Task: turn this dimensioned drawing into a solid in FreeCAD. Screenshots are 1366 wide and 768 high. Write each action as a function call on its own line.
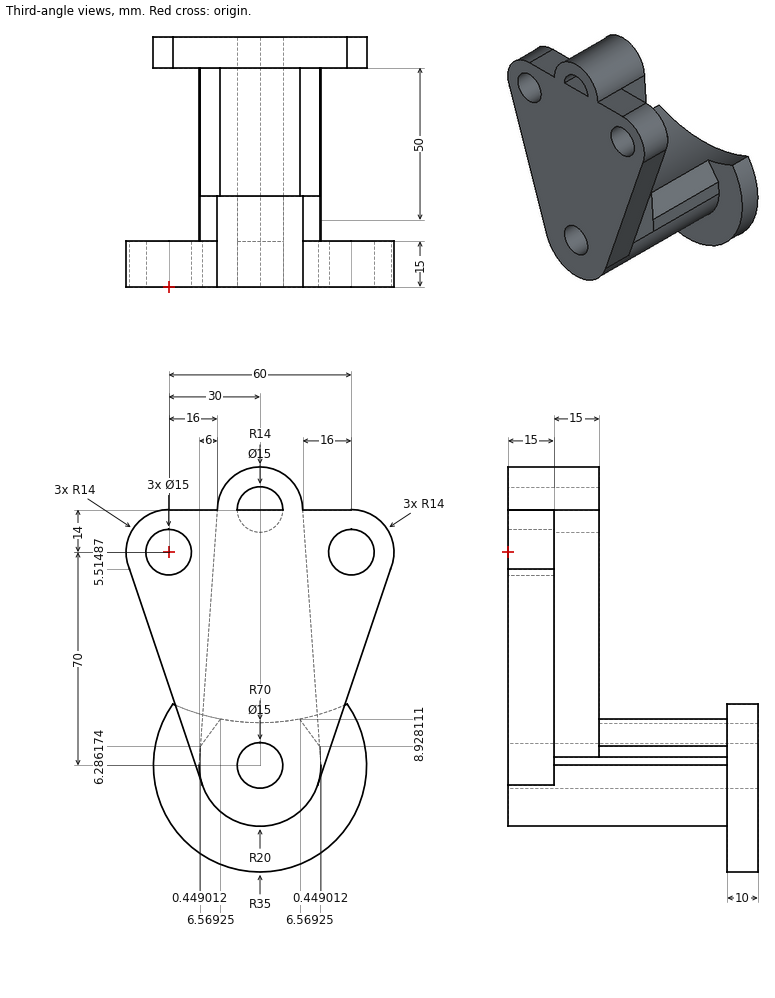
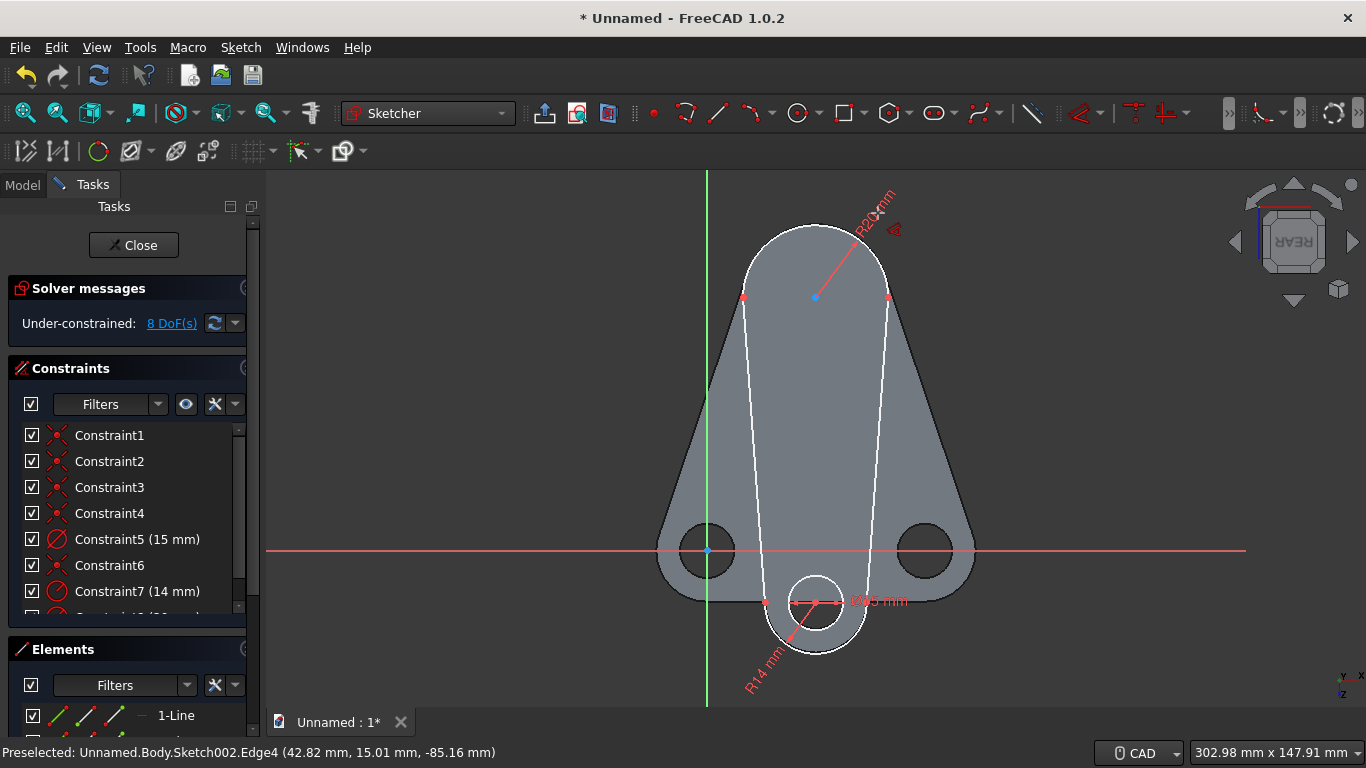
scroll(750, 390, up, 4)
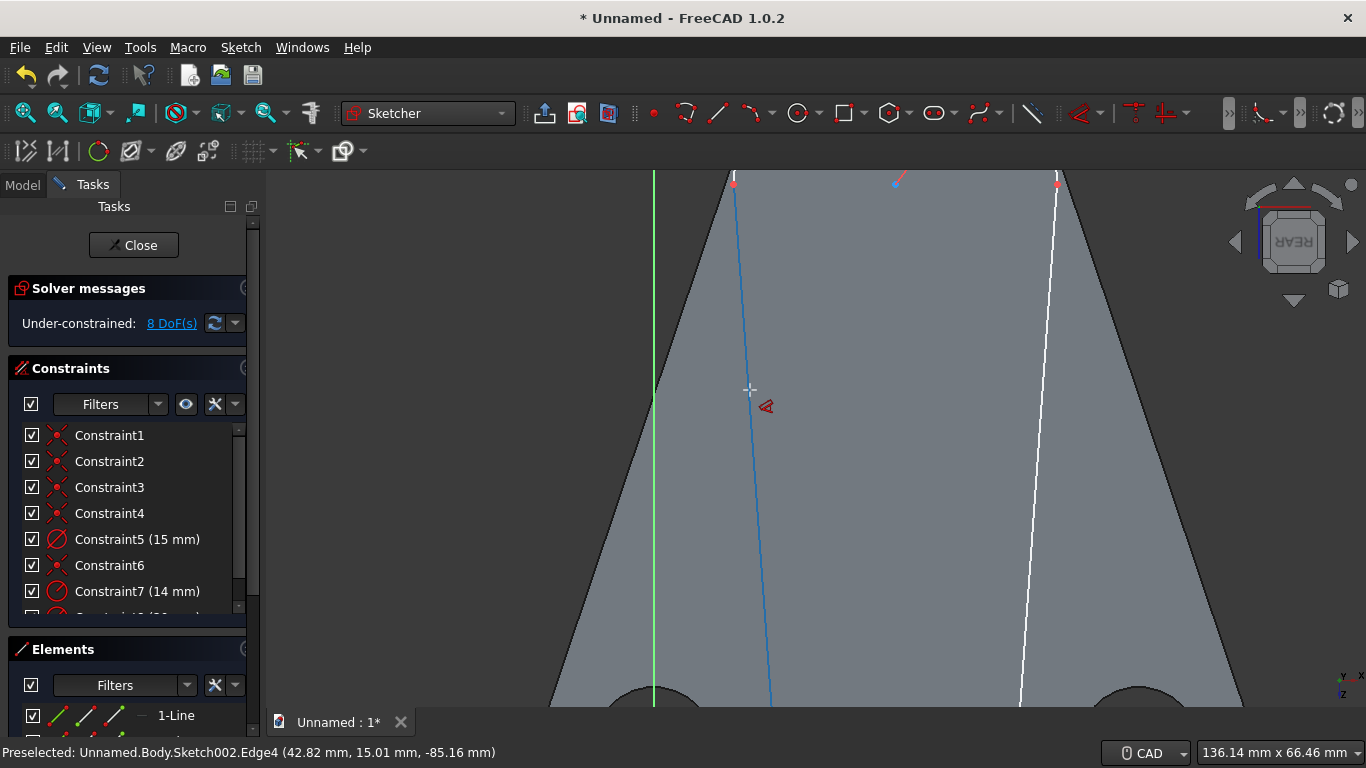
click(749, 388)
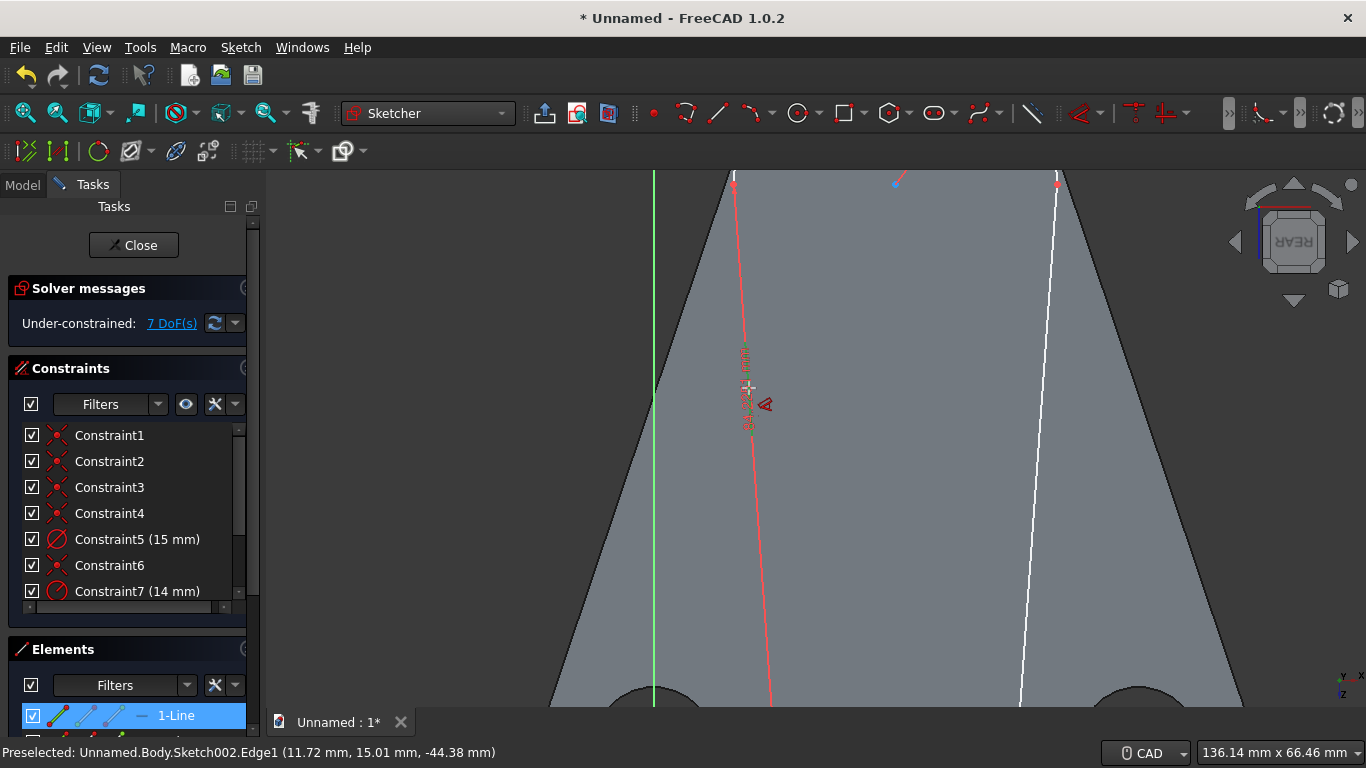
key(Escape)
key(Escape)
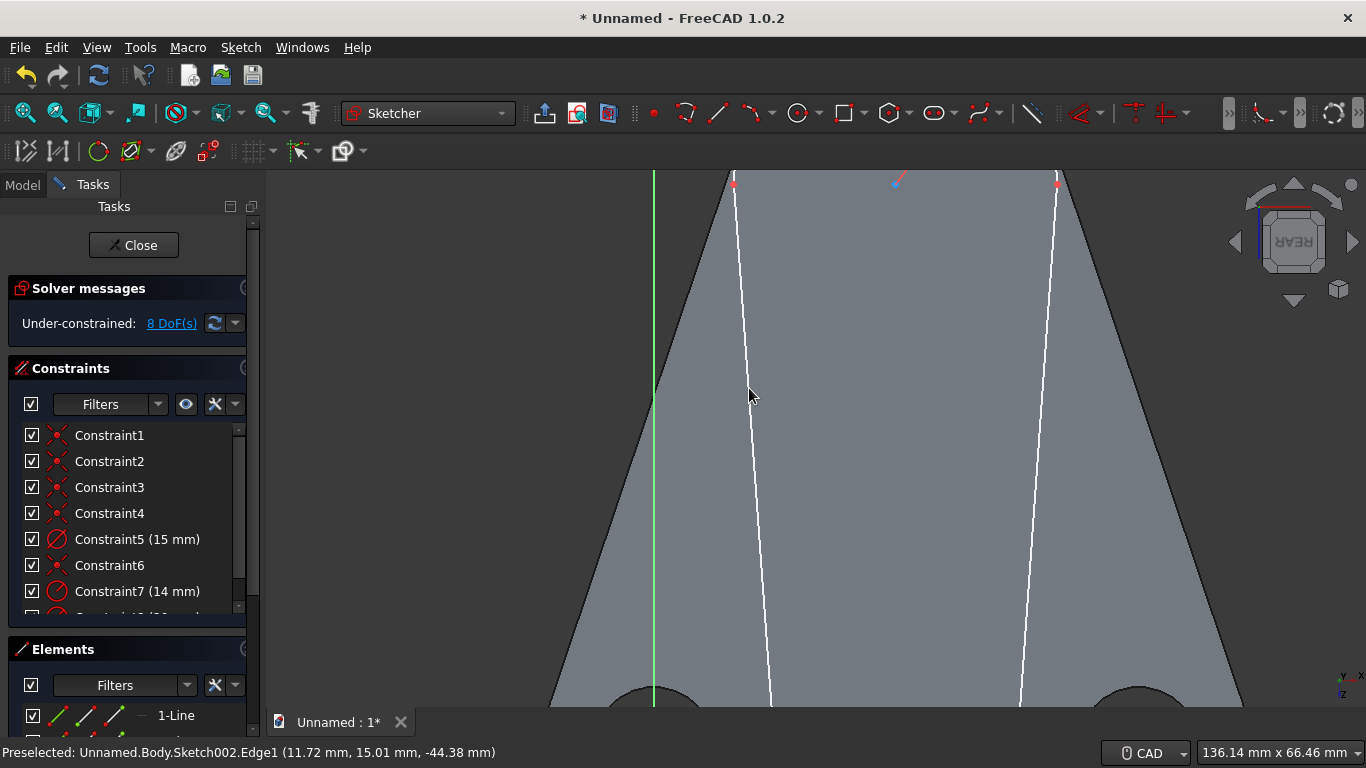
click(749, 388)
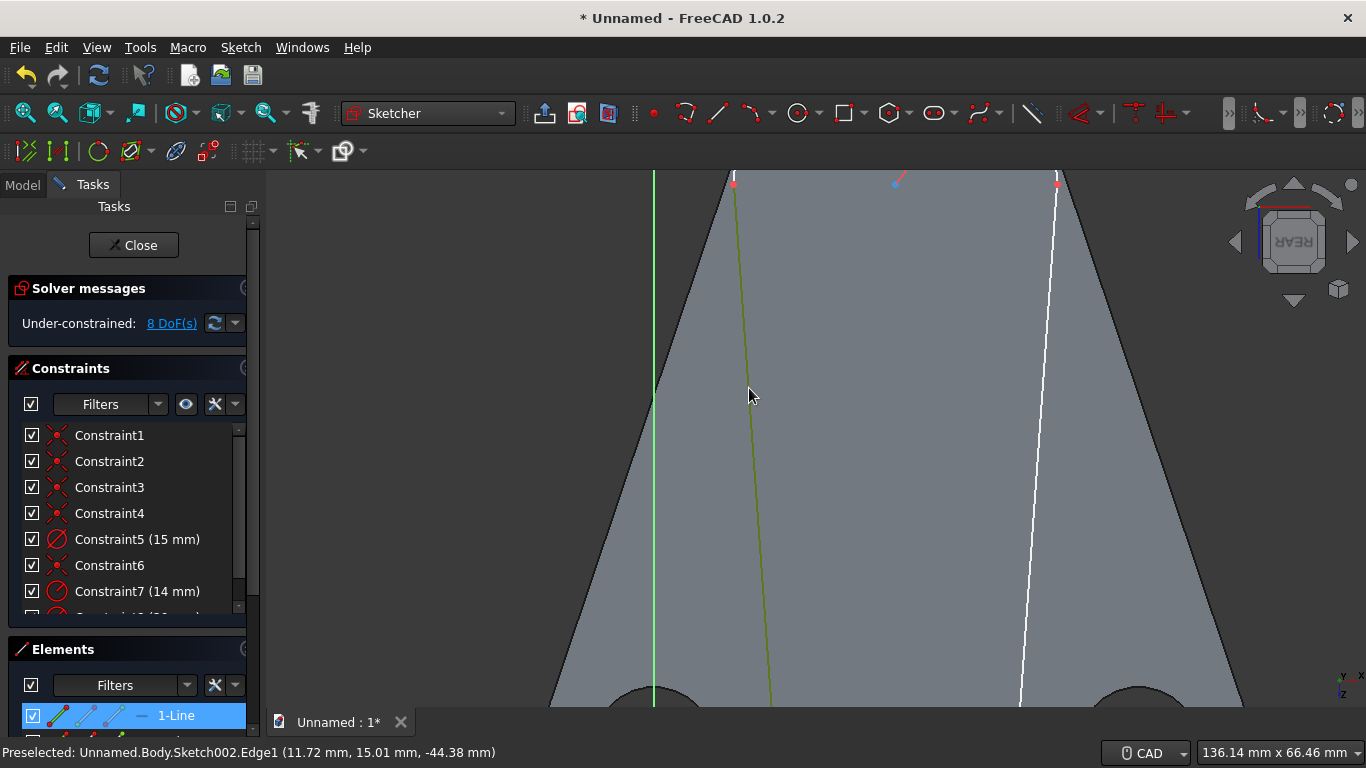
key(l)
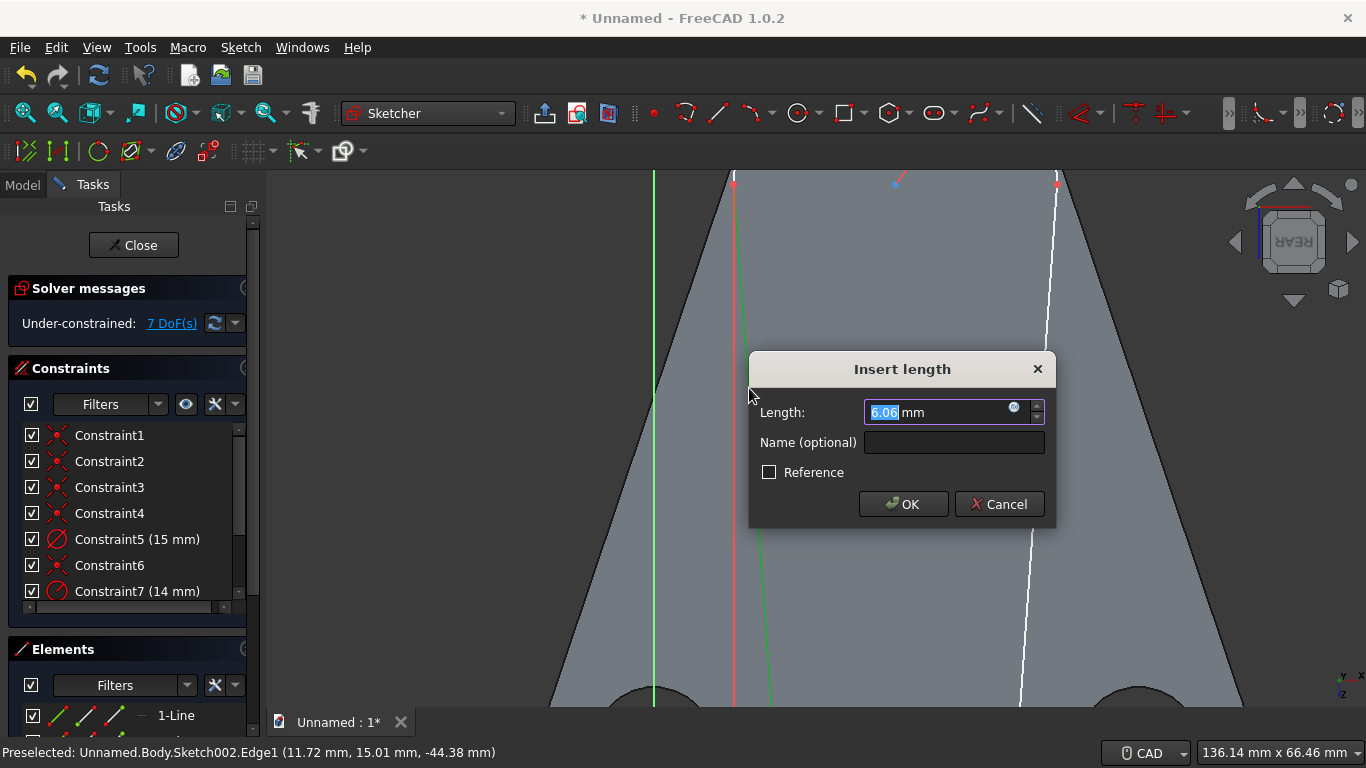
text(6)
key(Return)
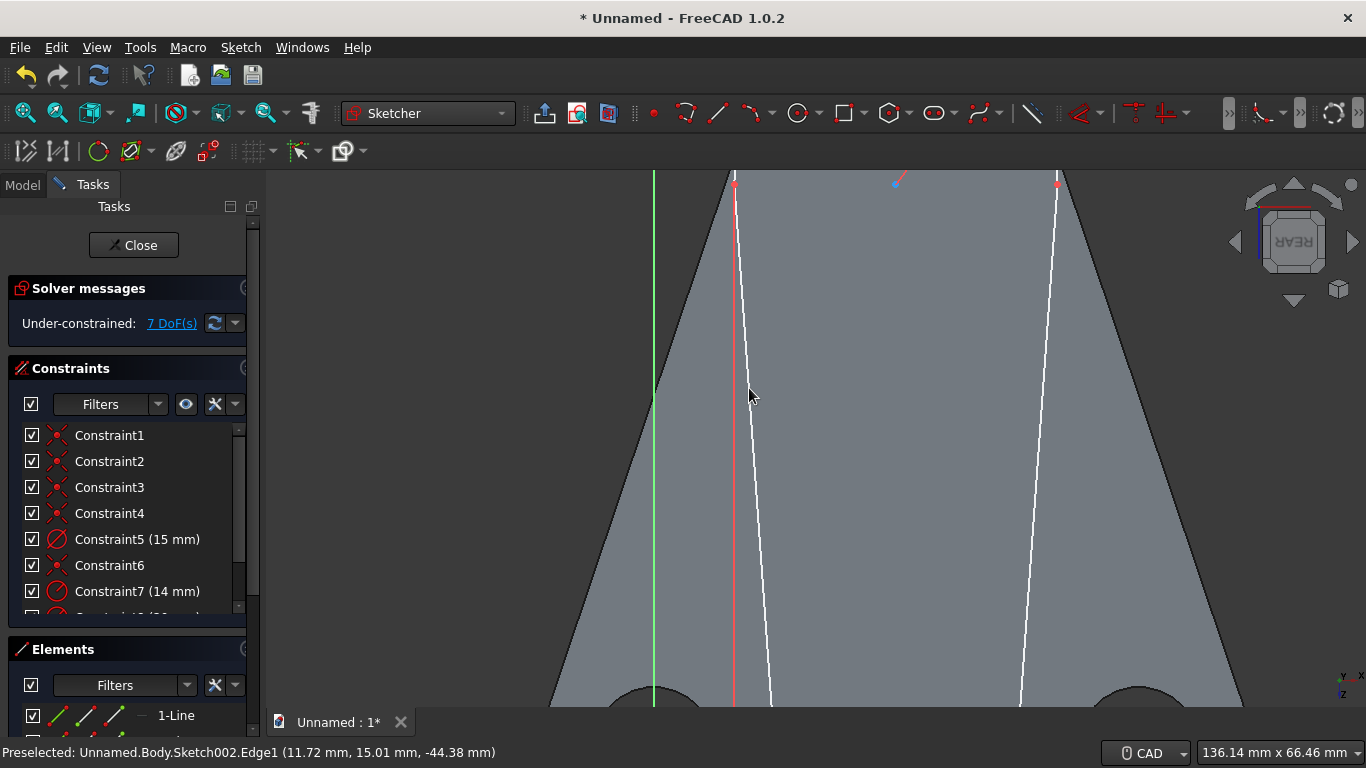
scroll(684, 404, down, 5)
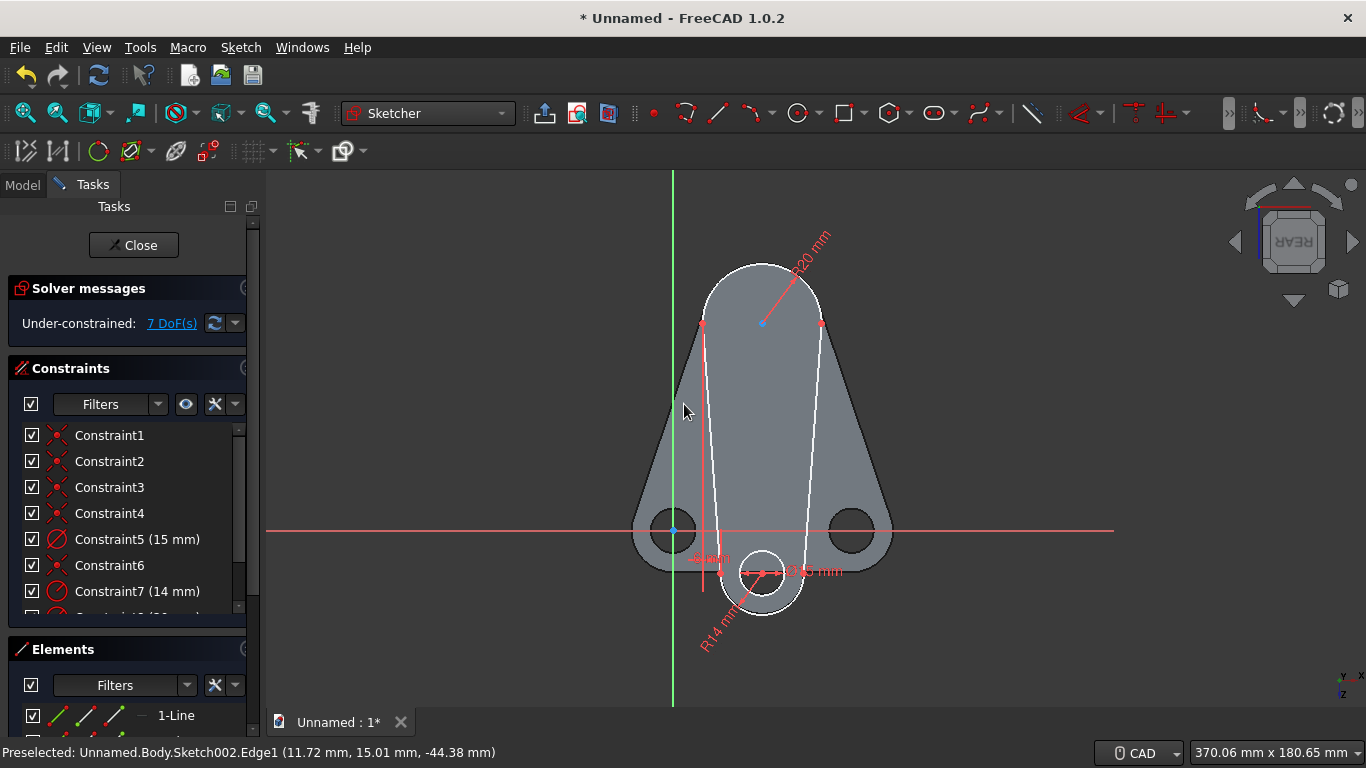
click(762, 573)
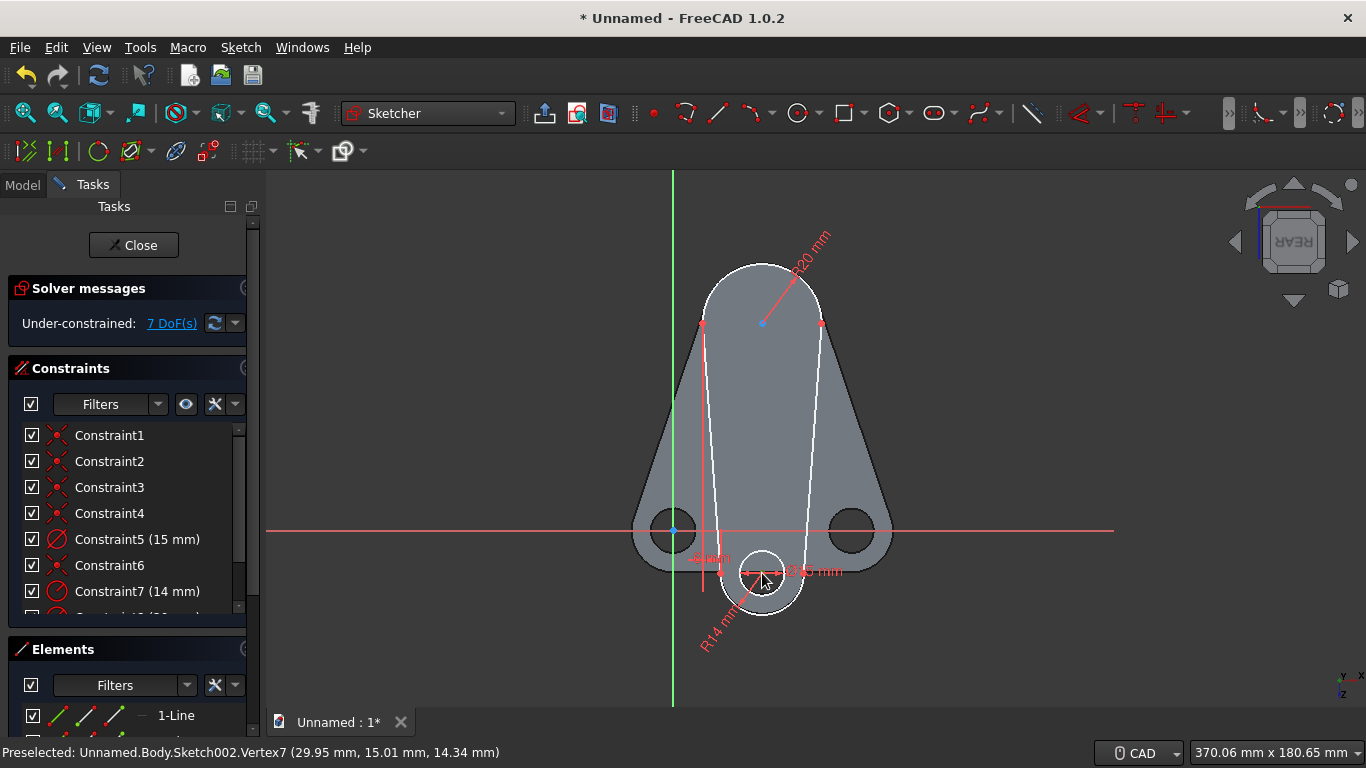
click(1102, 114)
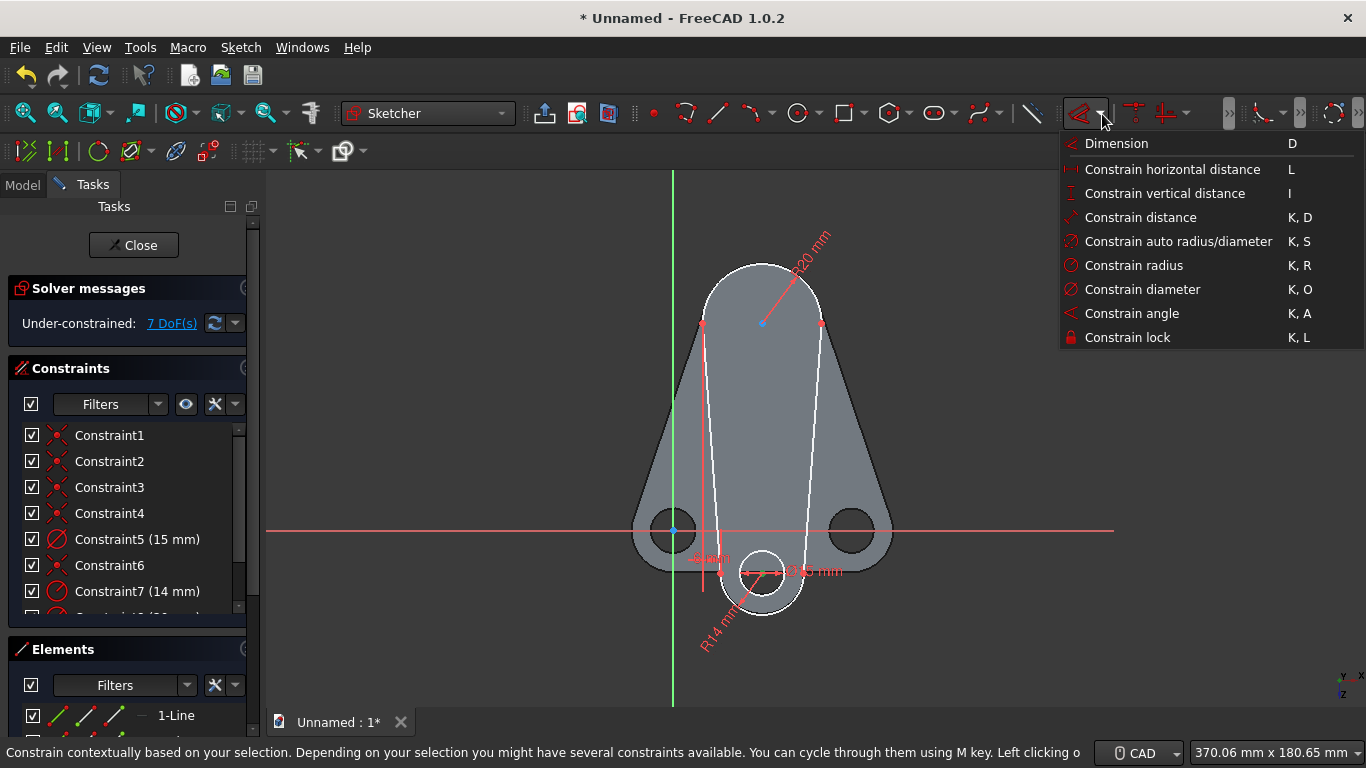
click(1212, 169)